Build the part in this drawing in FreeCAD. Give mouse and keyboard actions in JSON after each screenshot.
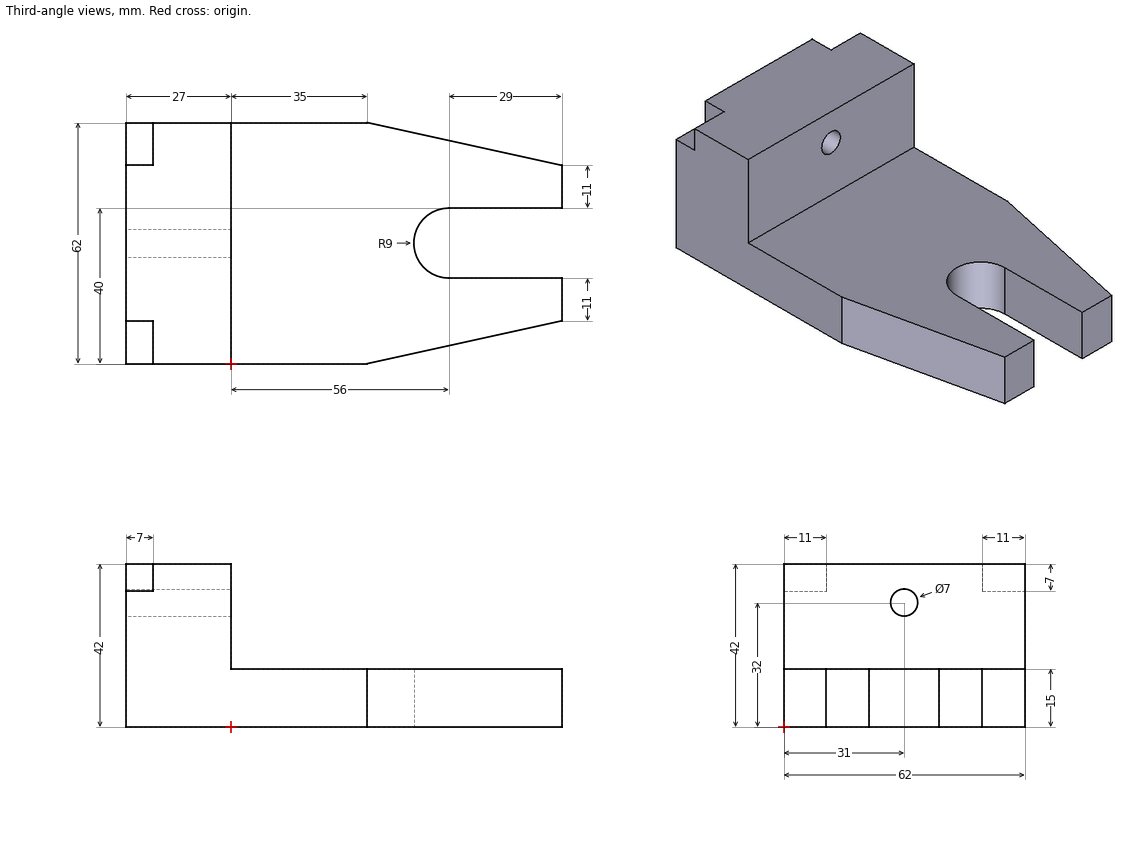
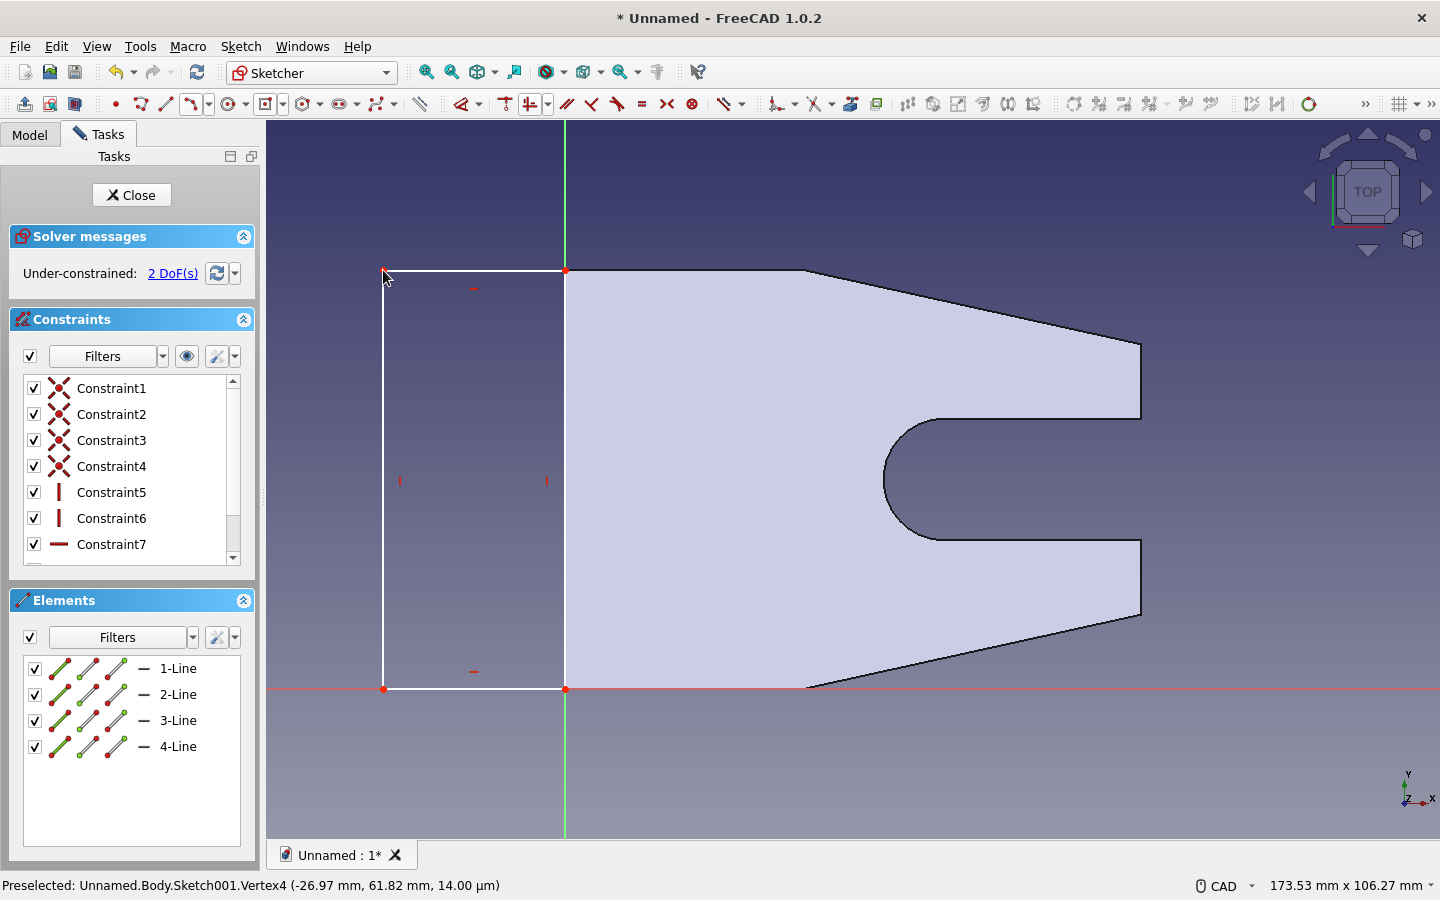
{"action": "left_click", "coordinate": [460, 104]}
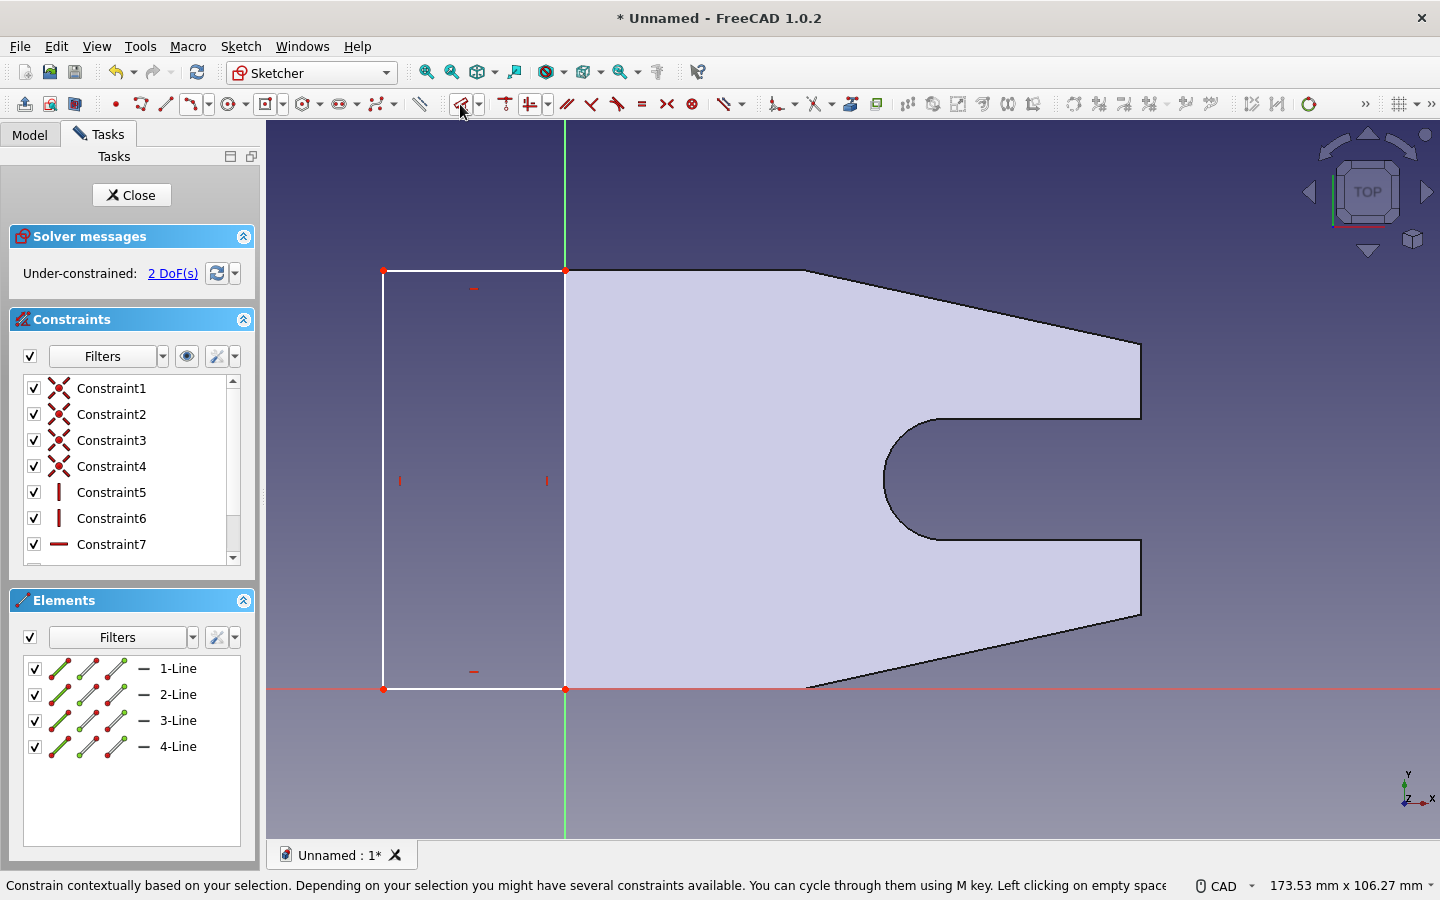
{"action": "left_click", "coordinate": [565, 564]}
{"action": "left_click", "coordinate": [599, 480]}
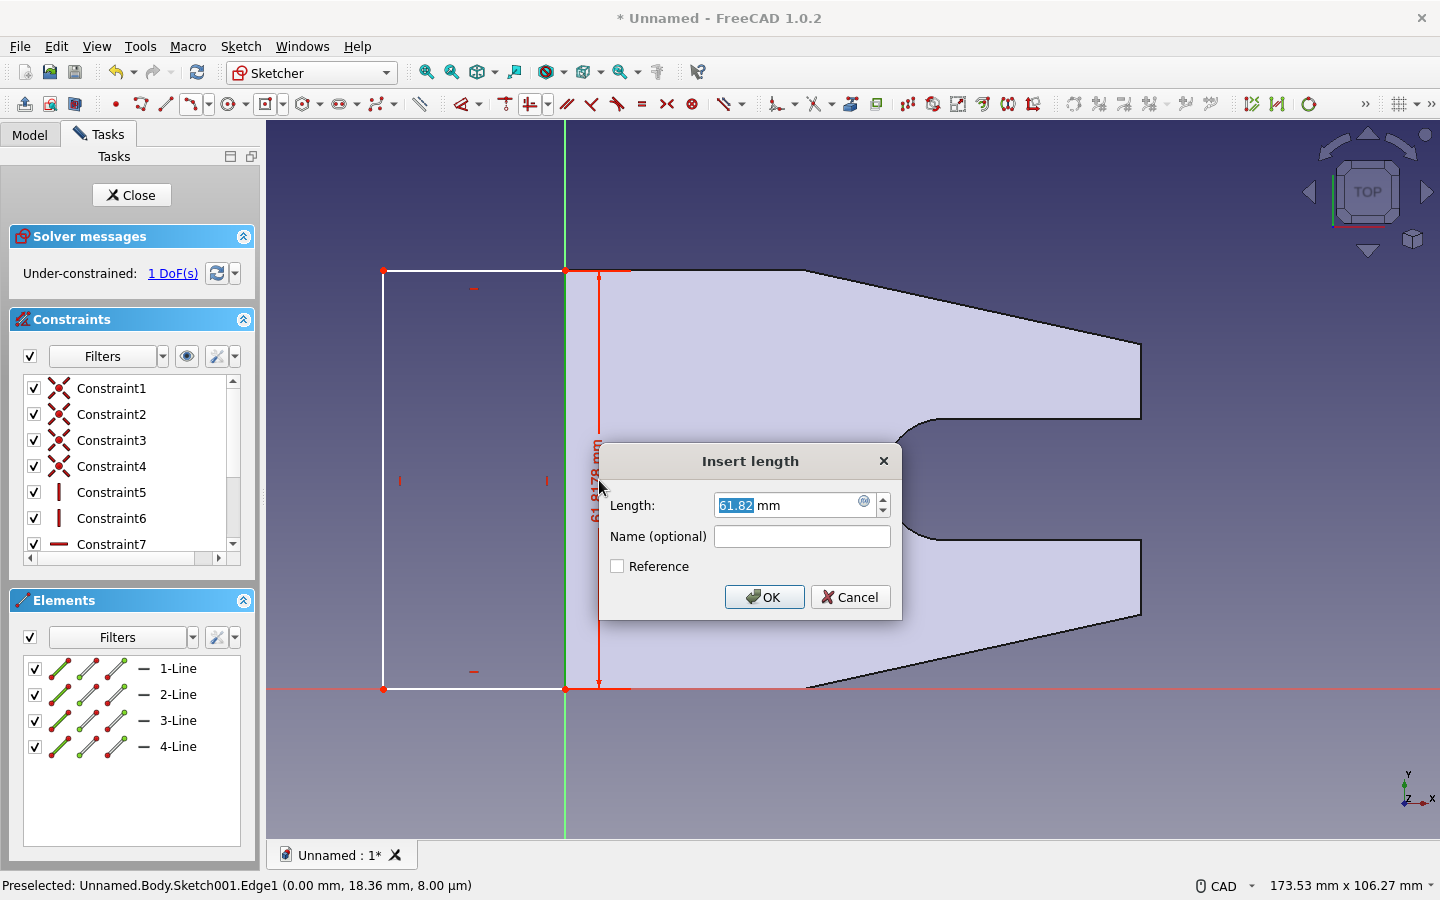
{"action": "type", "text": "62"}
{"action": "key", "text": "Return"}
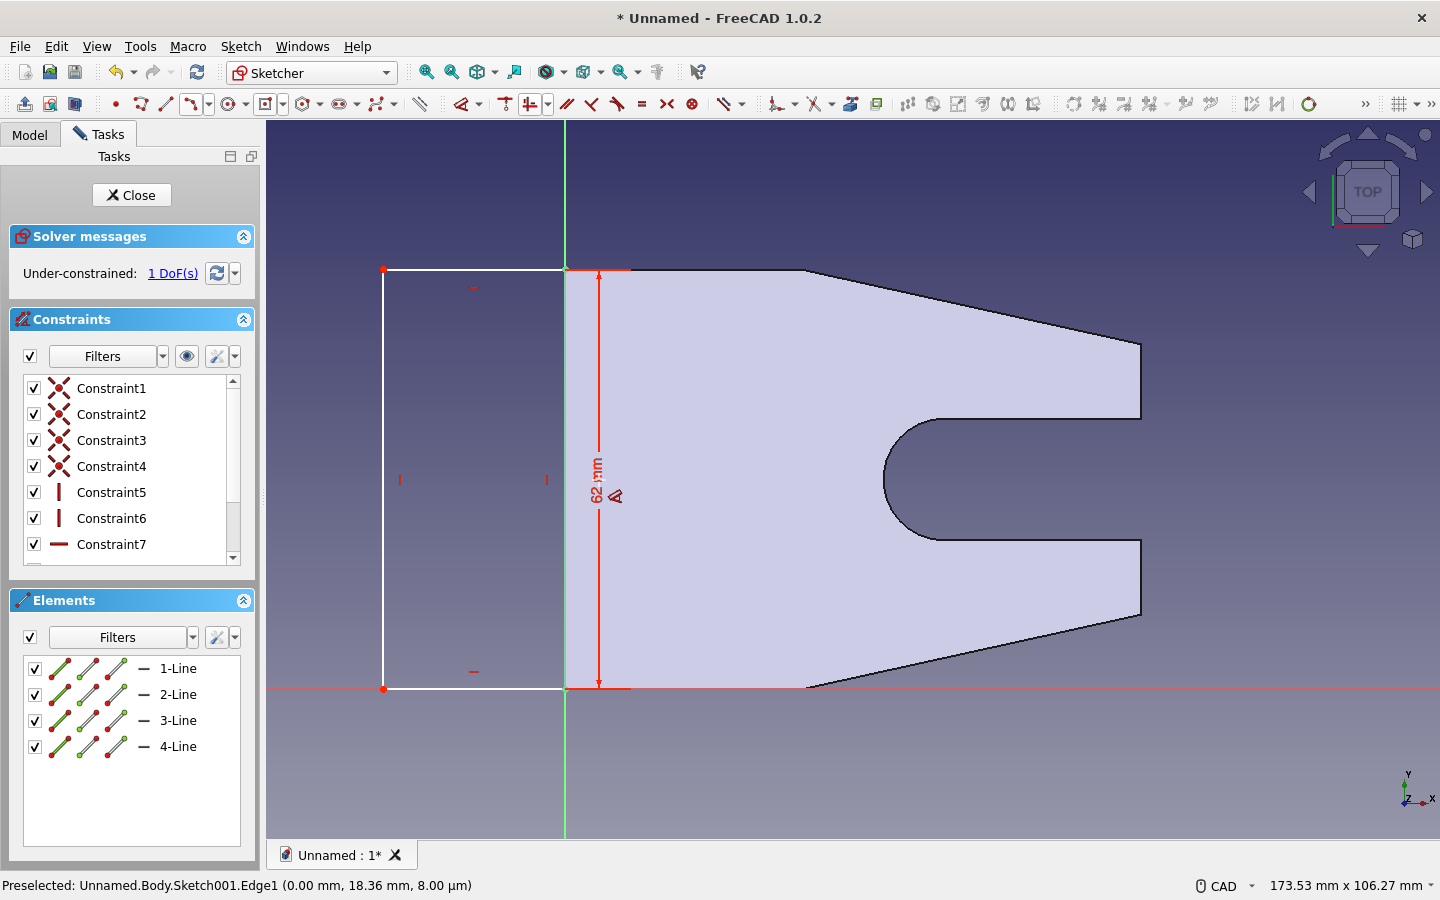
{"action": "left_click", "coordinate": [511, 270]}
{"action": "left_click", "coordinate": [474, 236]}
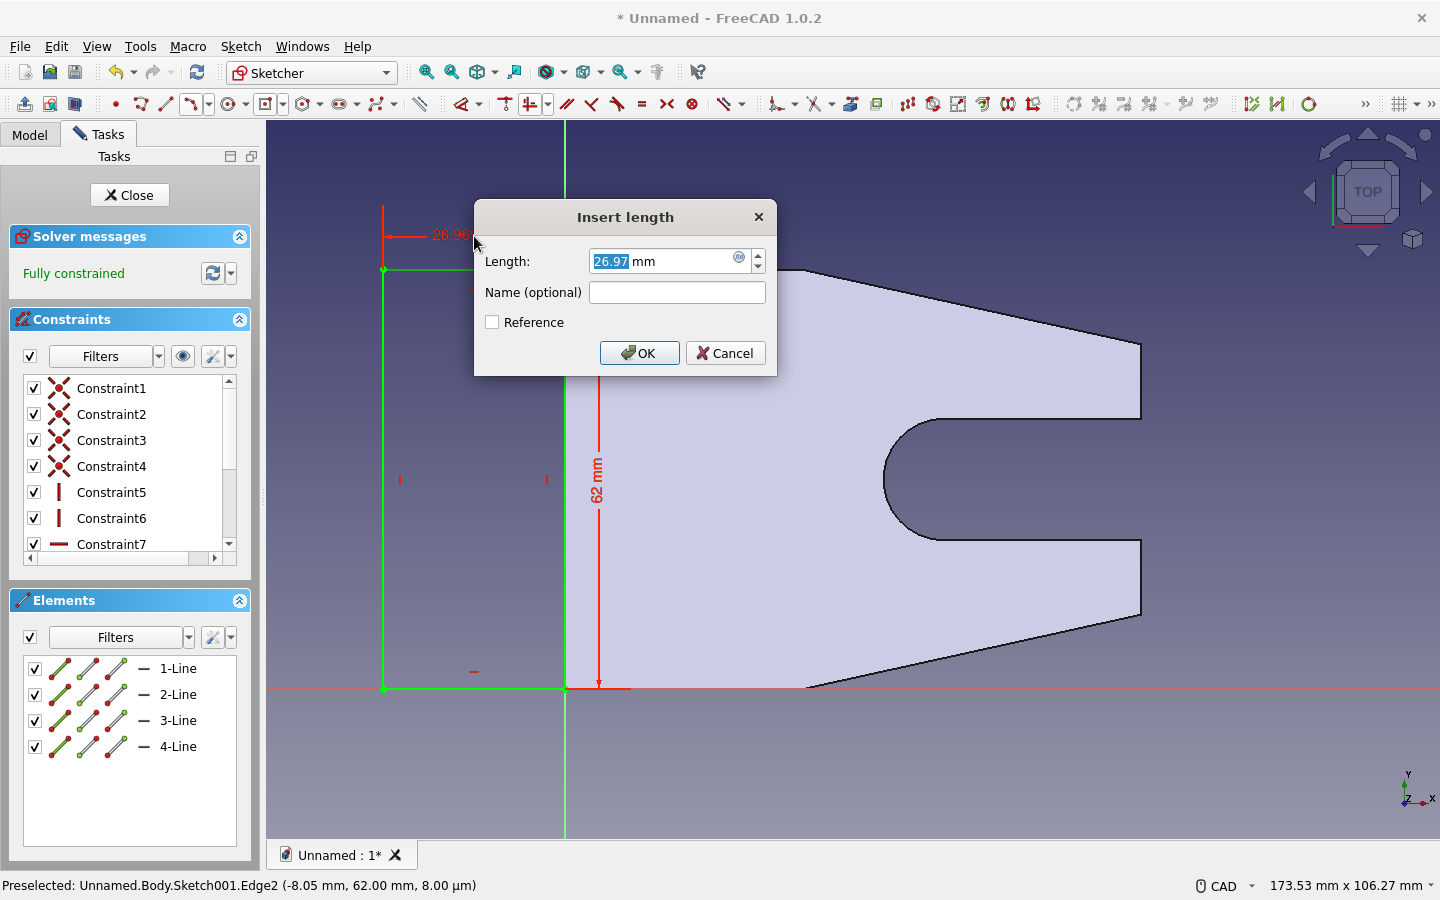
{"action": "type", "text": "27"}
{"action": "key", "text": "Return"}
{"action": "key", "text": "Escape"}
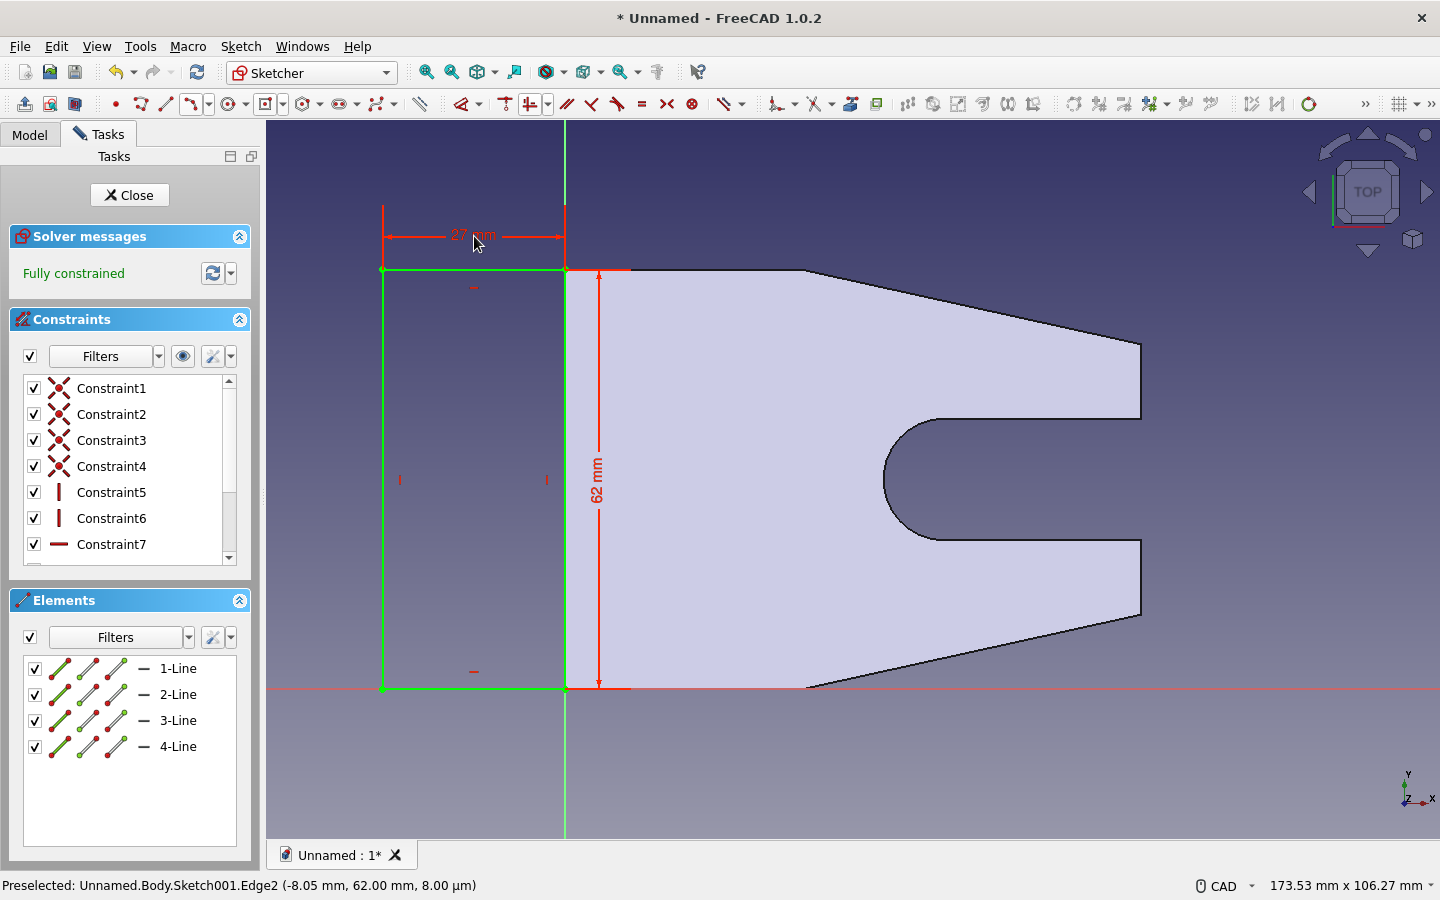
{"action": "left_click", "coordinate": [130, 195]}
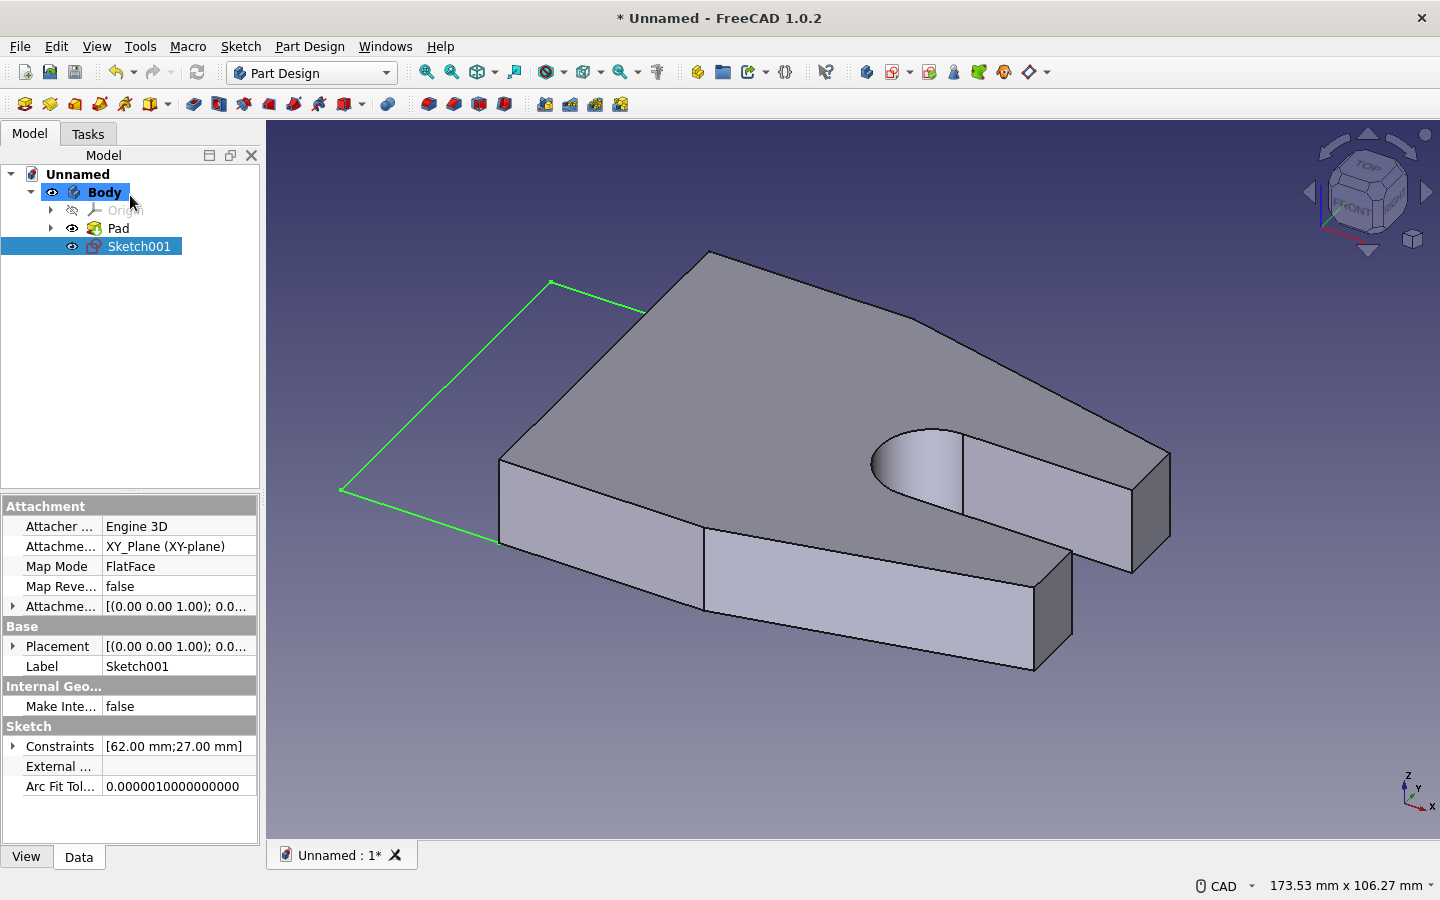
{"action": "left_click", "coordinate": [25, 104]}